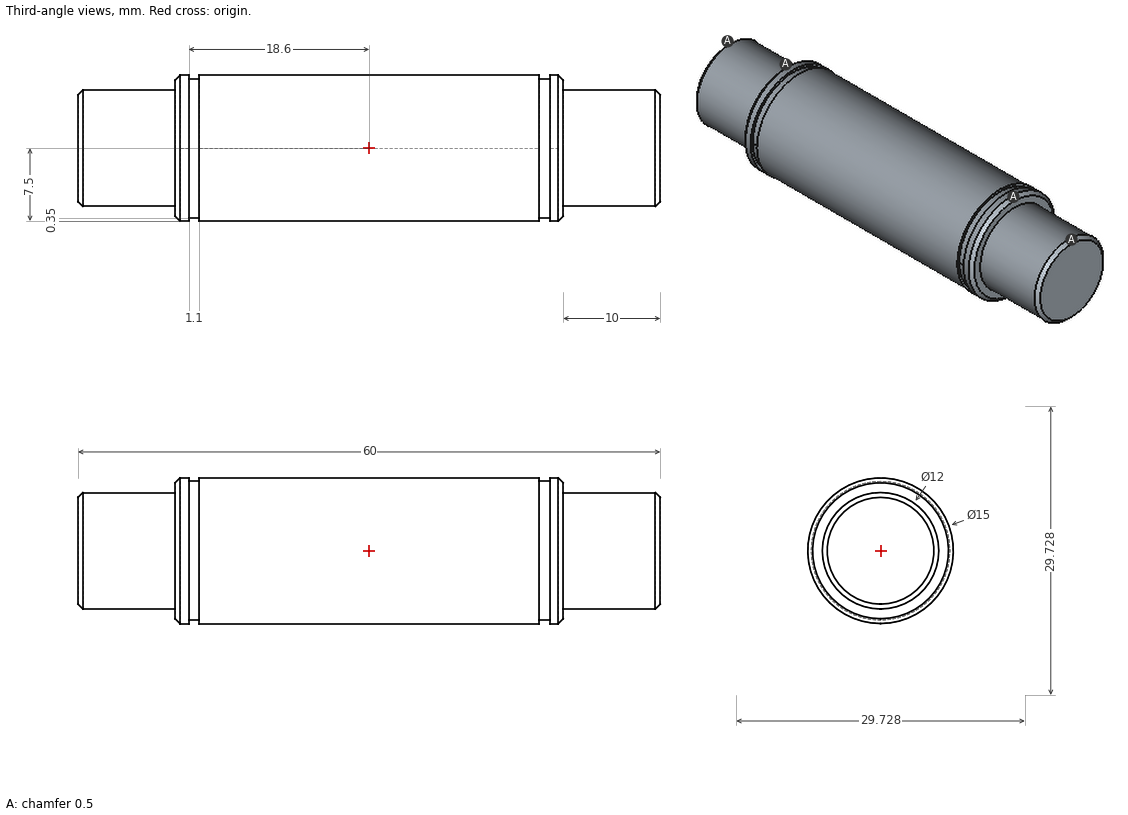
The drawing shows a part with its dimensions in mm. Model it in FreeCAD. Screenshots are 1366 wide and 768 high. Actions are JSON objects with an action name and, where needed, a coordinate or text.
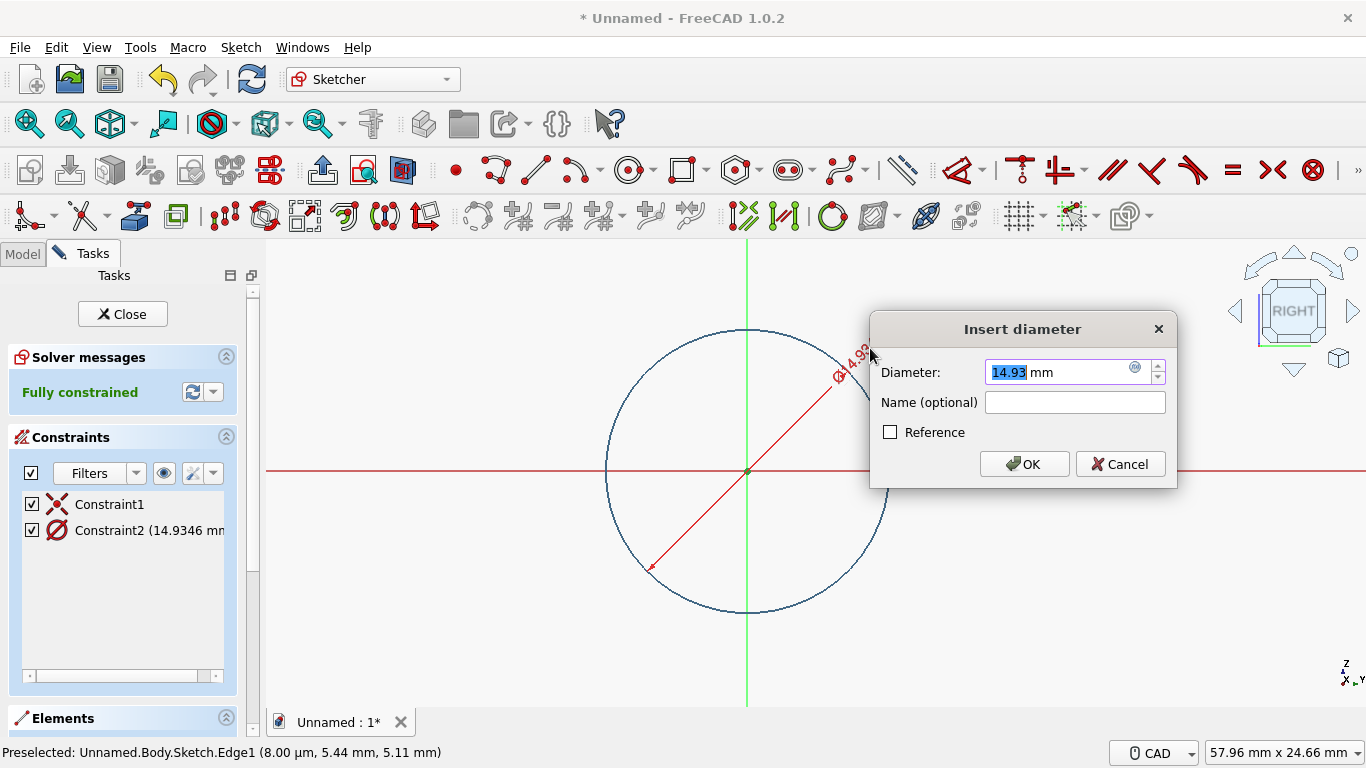
{"action": "type", "text": "15"}
{"action": "key", "text": "Return"}
{"action": "key", "text": "Escape"}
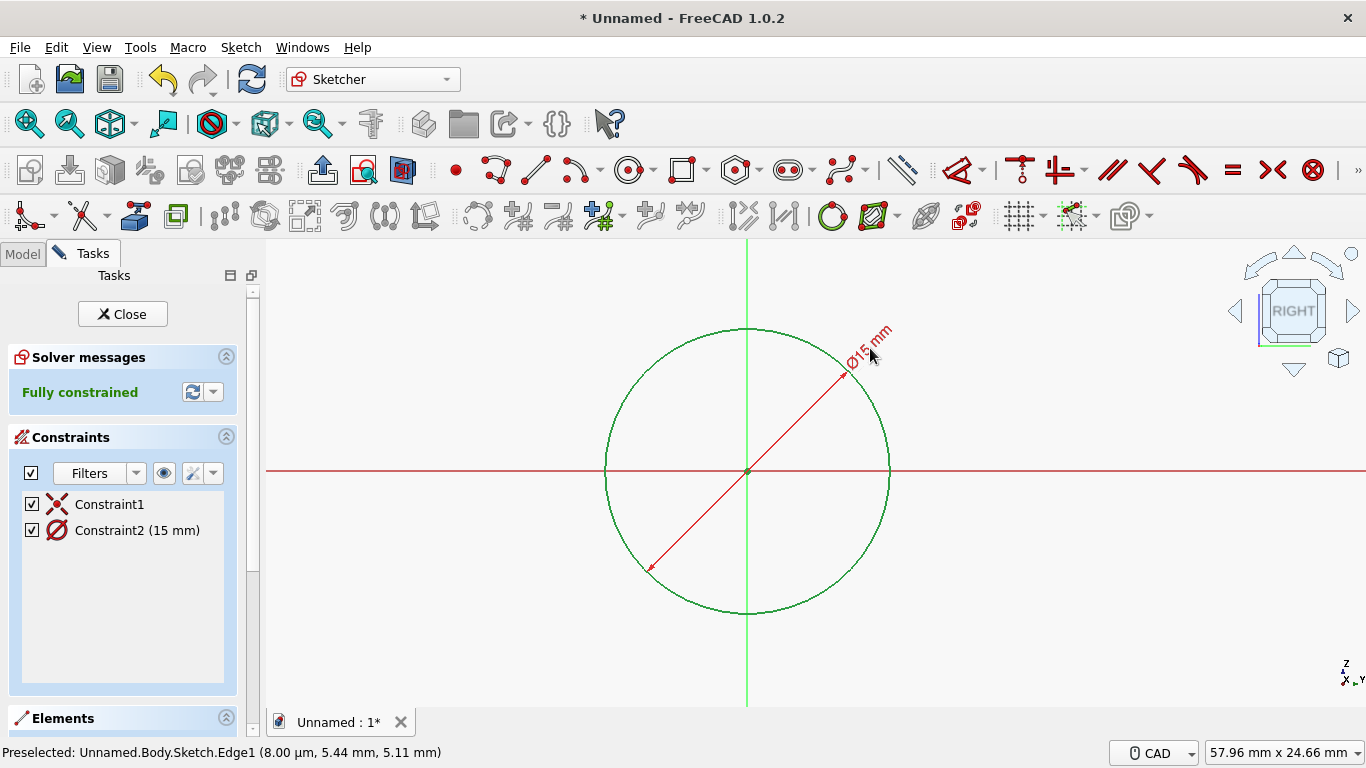
{"action": "left_click", "coordinate": [123, 314]}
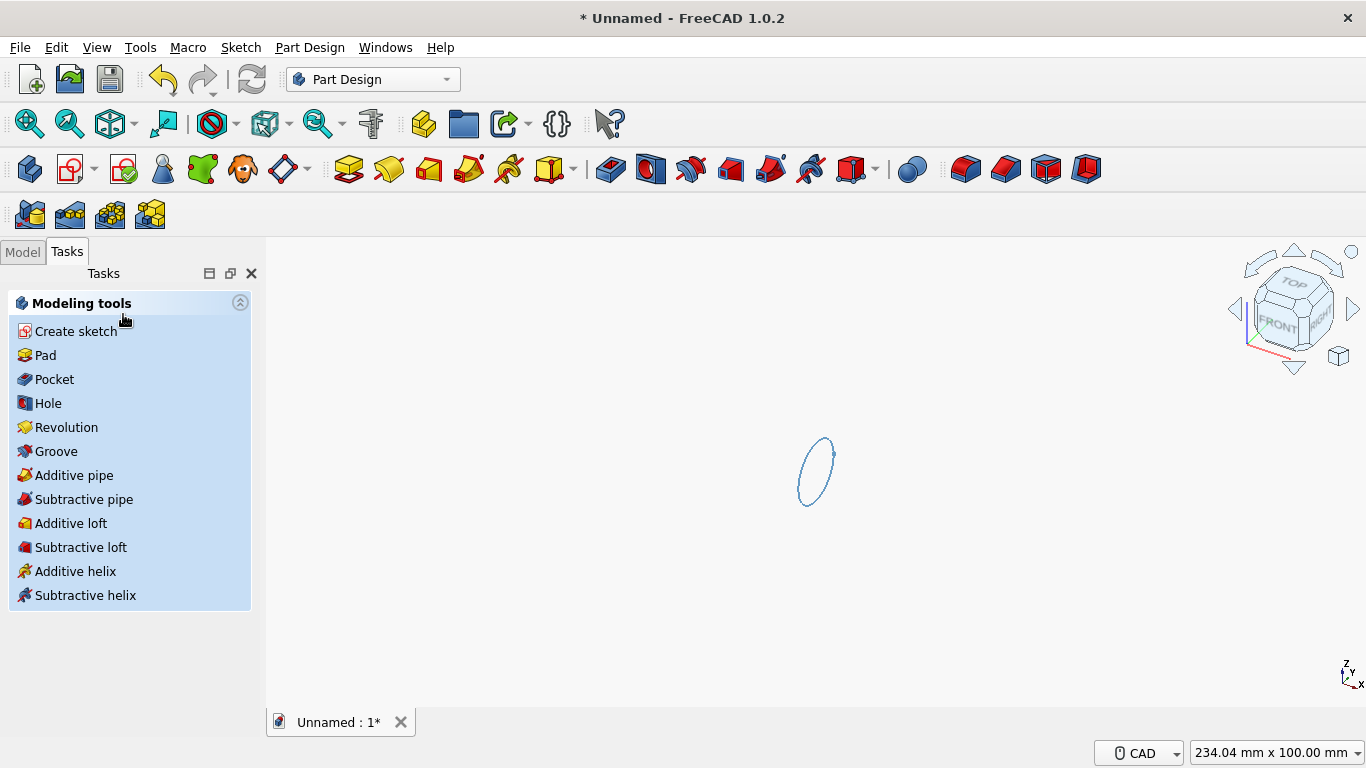
{"action": "left_click", "coordinate": [350, 170]}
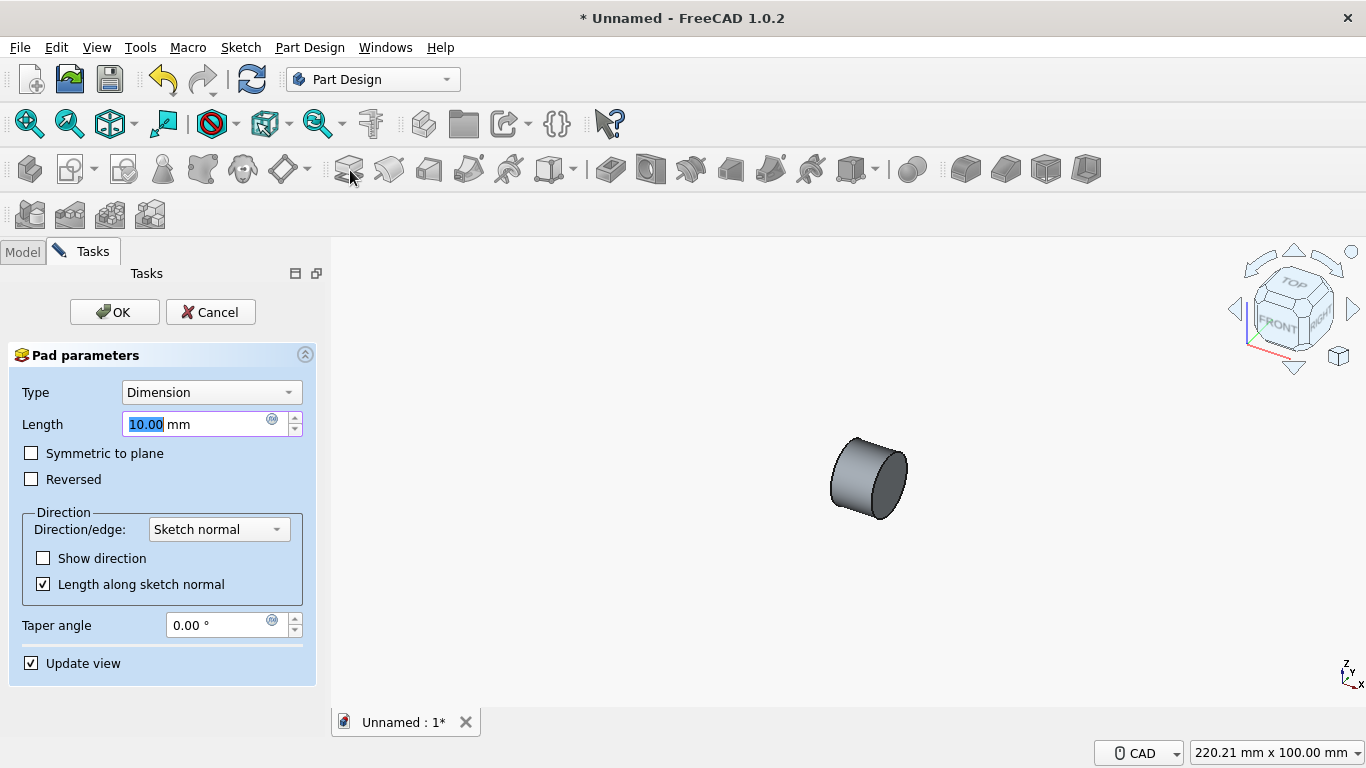
{"action": "type", "text": "60"}
{"action": "key", "text": "Tab"}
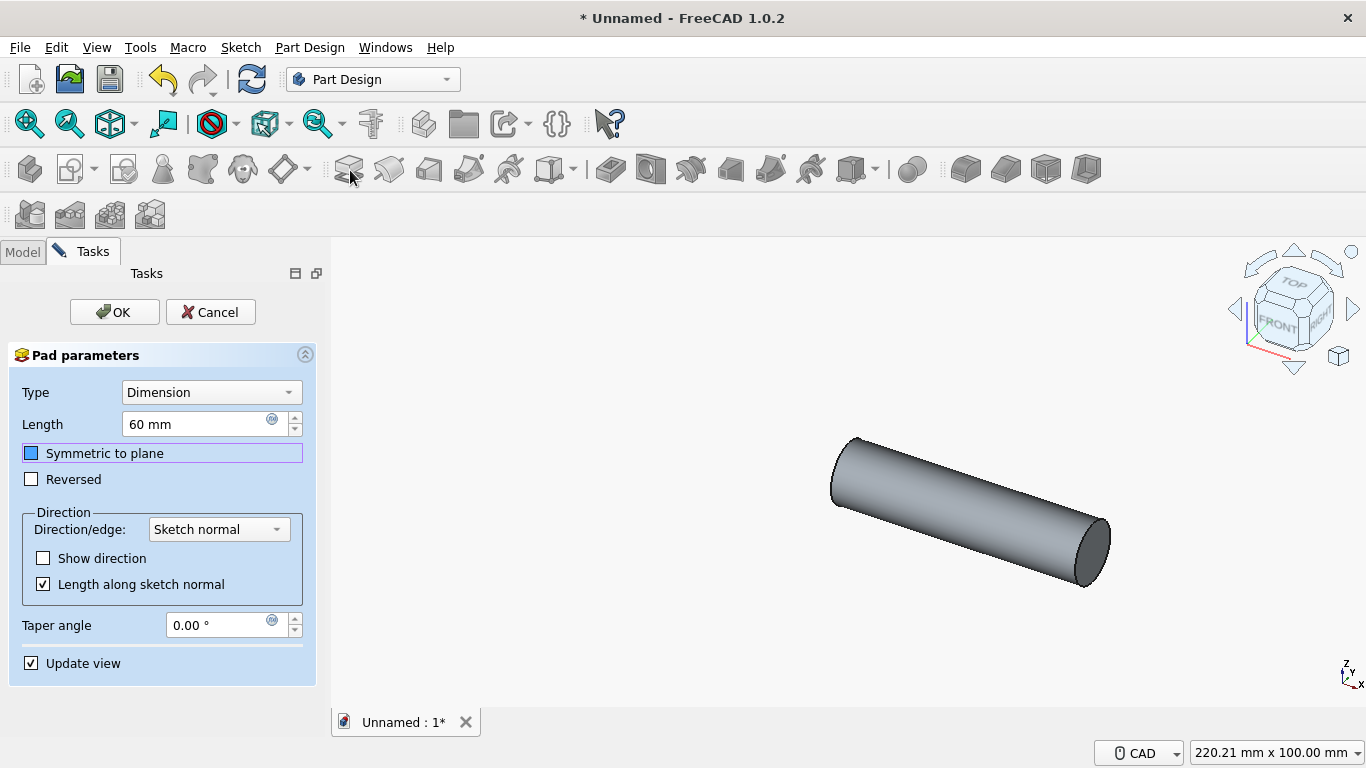
{"action": "left_click", "coordinate": [30, 453]}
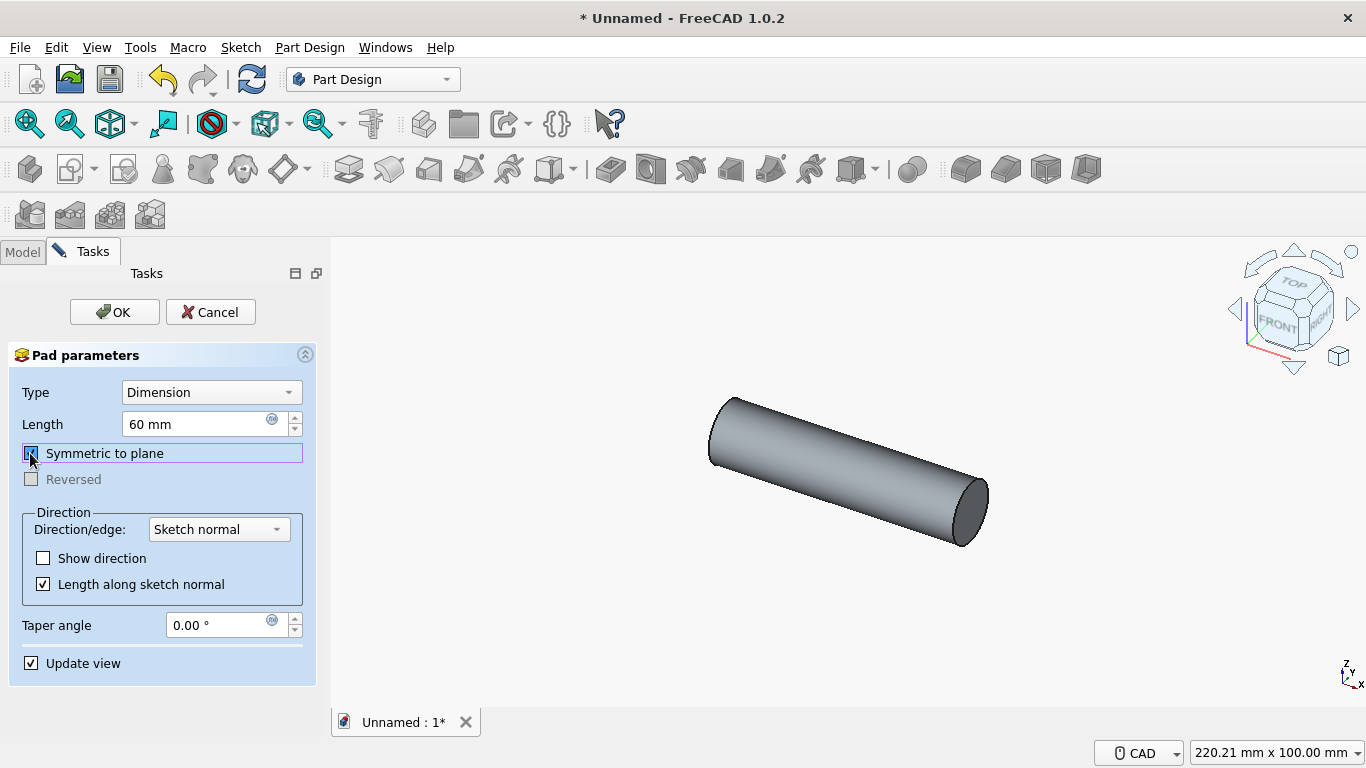
{"action": "left_click", "coordinate": [115, 312]}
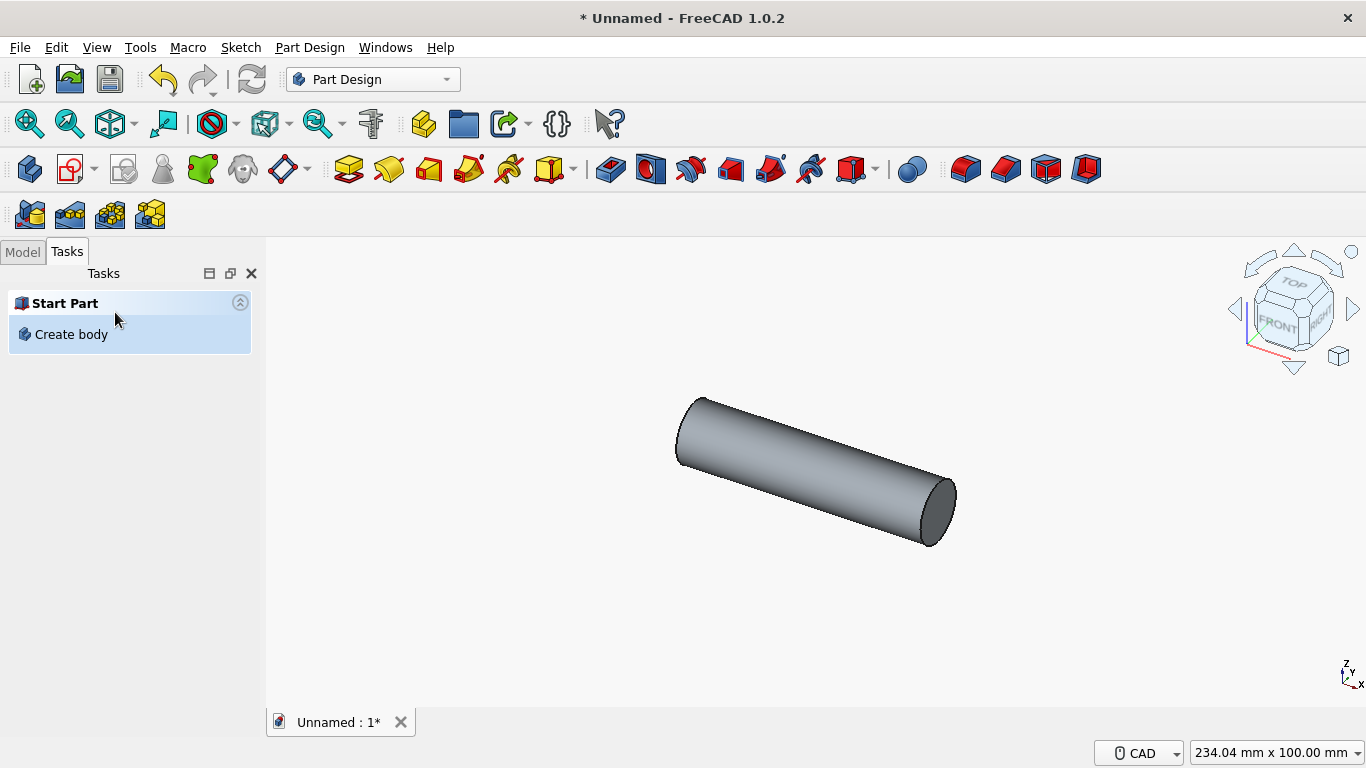
{"action": "key", "text": "v f"}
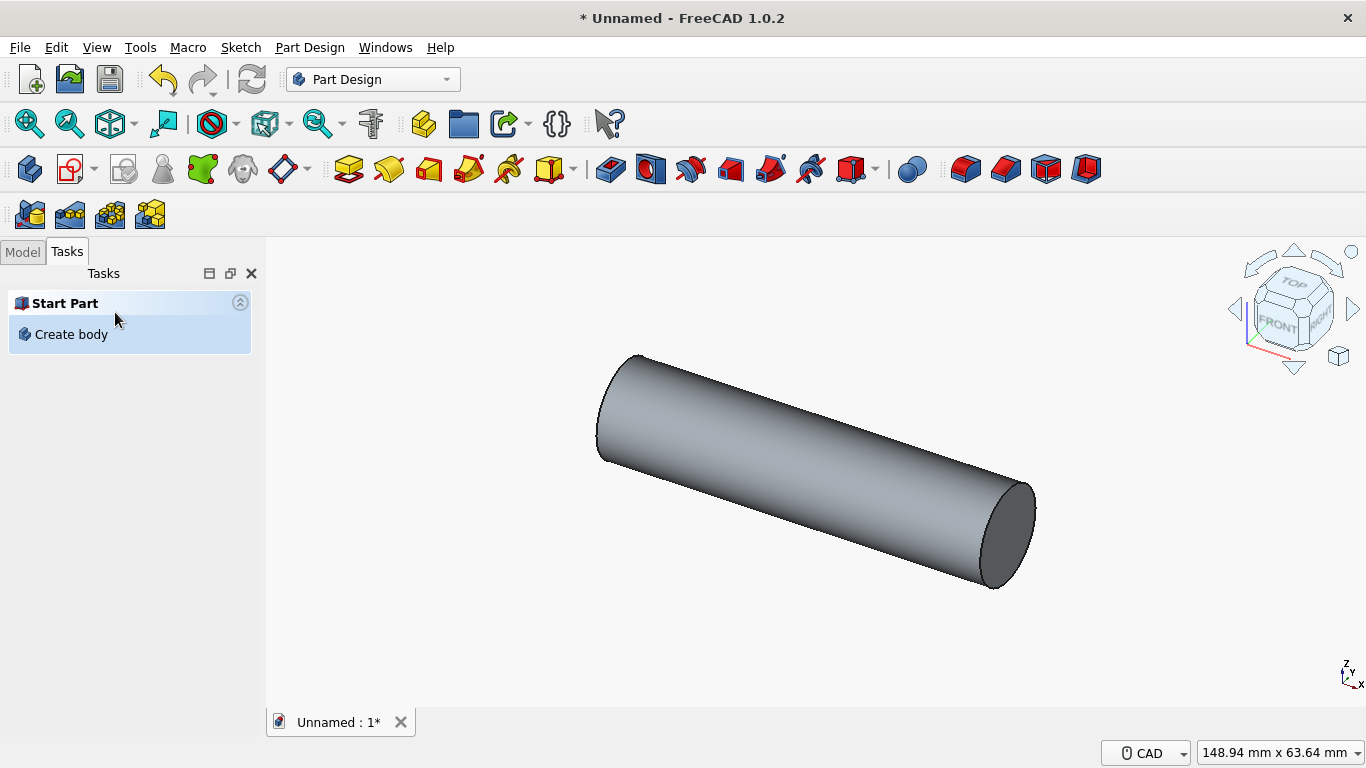
{"action": "left_click", "coordinate": [1008, 535]}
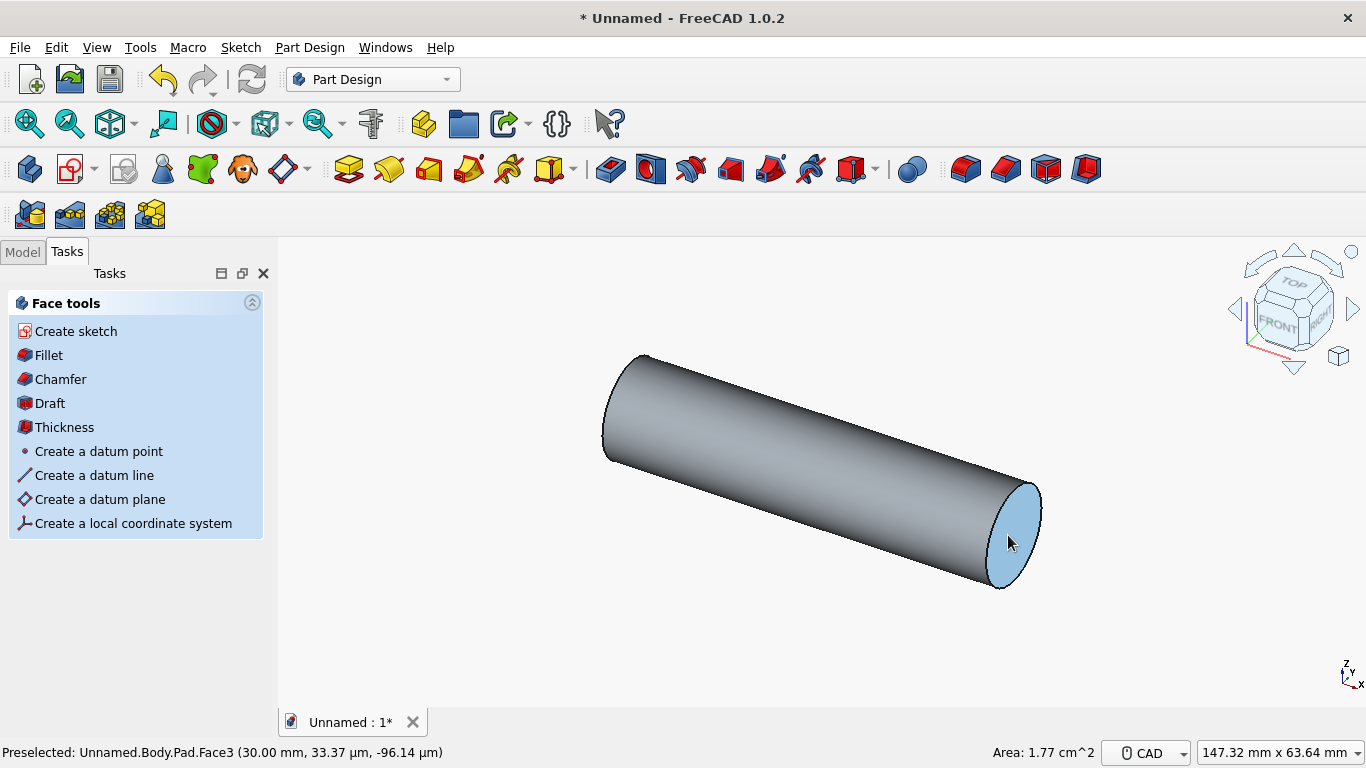
{"action": "left_click", "coordinate": [70, 170]}